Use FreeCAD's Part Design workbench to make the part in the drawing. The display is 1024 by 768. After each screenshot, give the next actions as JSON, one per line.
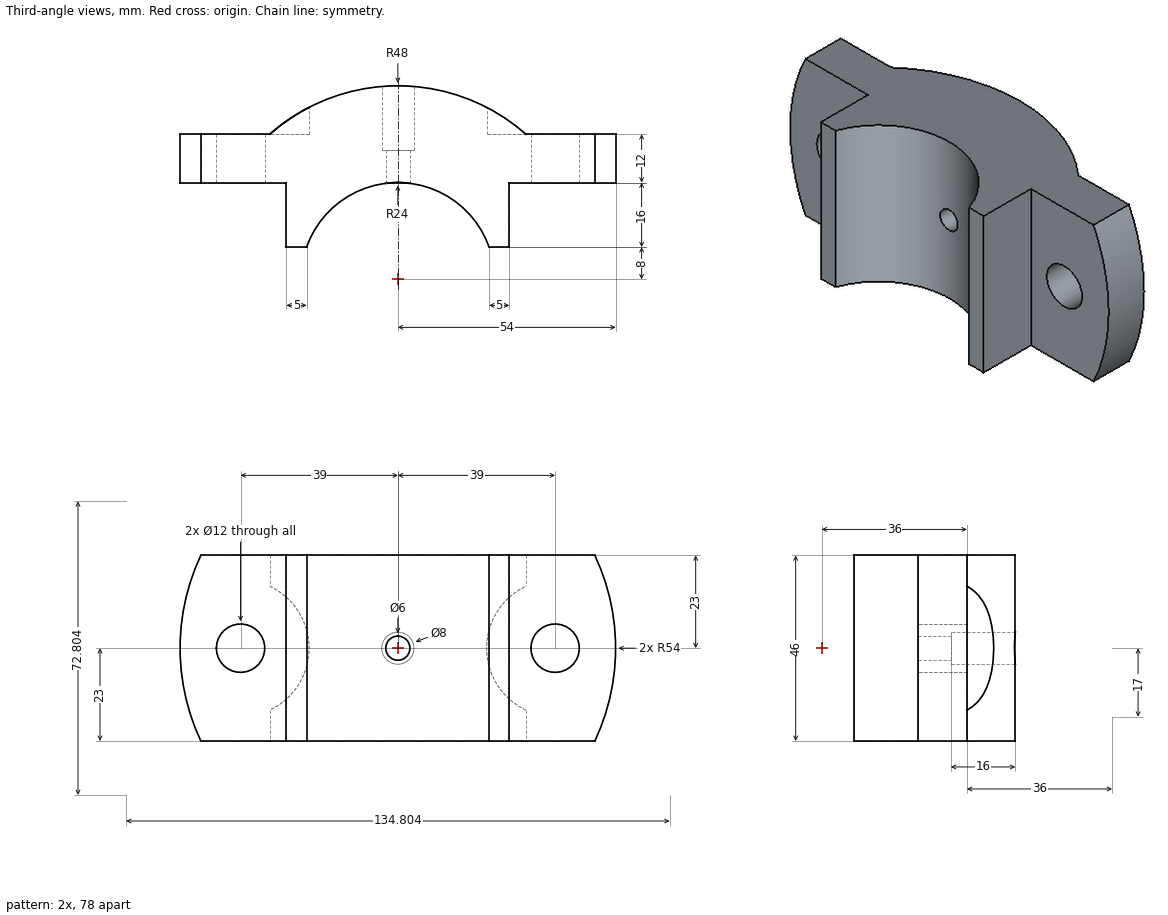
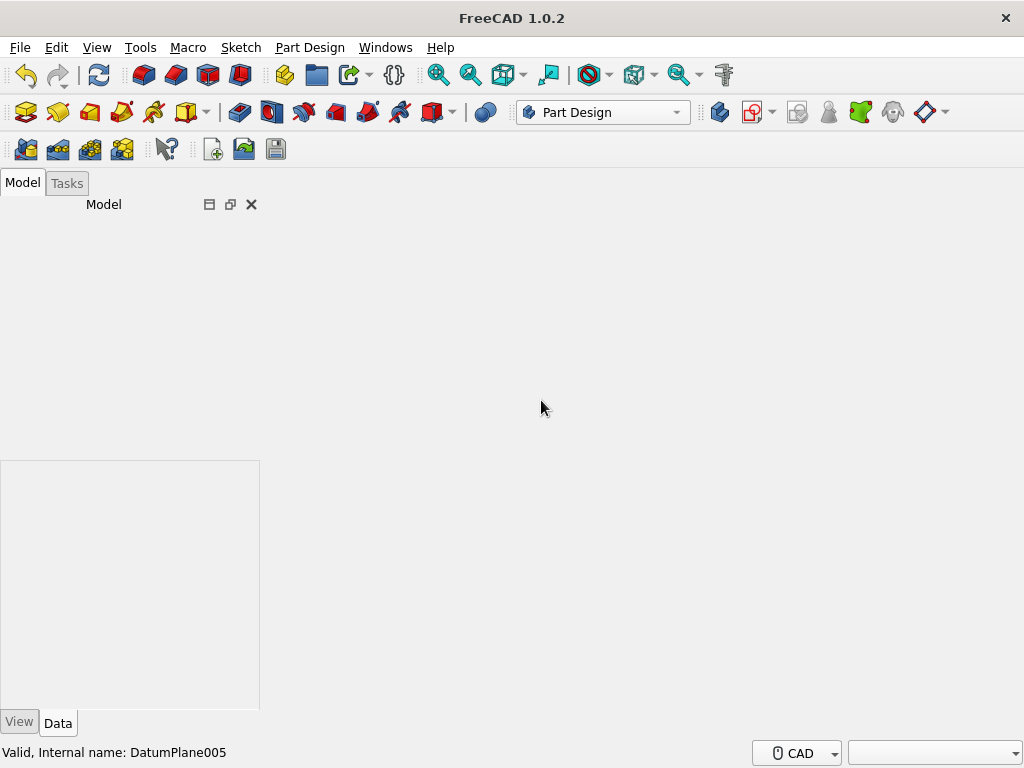
{"action": "left_click", "coordinate": [212, 150]}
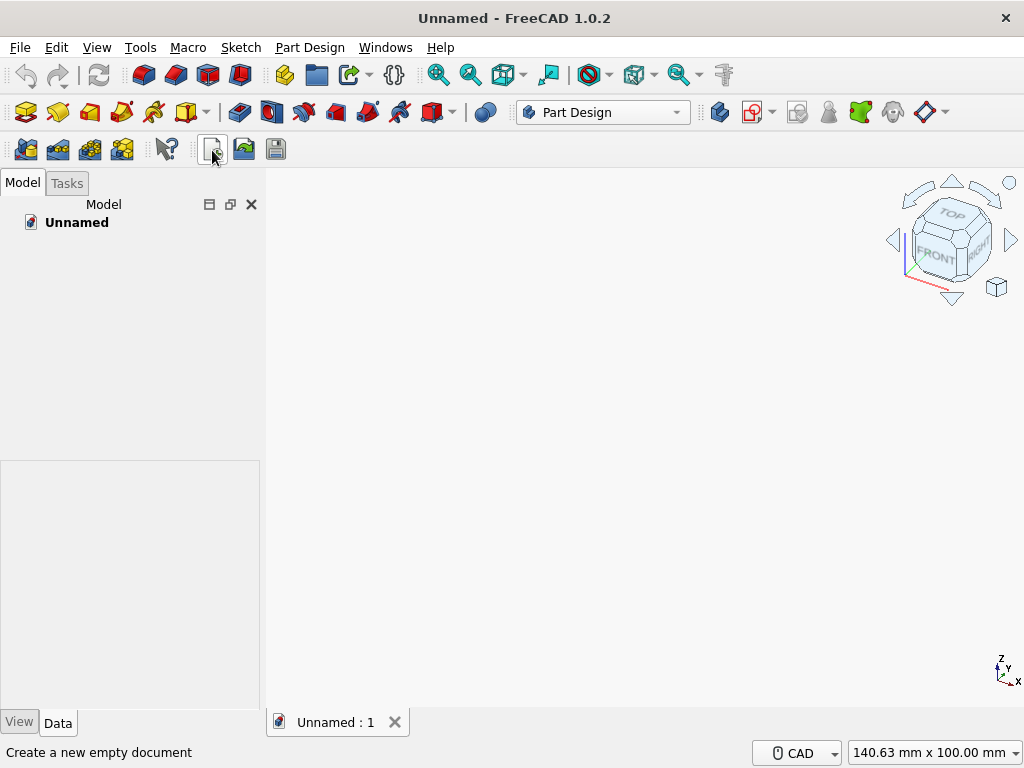
{"action": "left_click", "coordinate": [752, 112]}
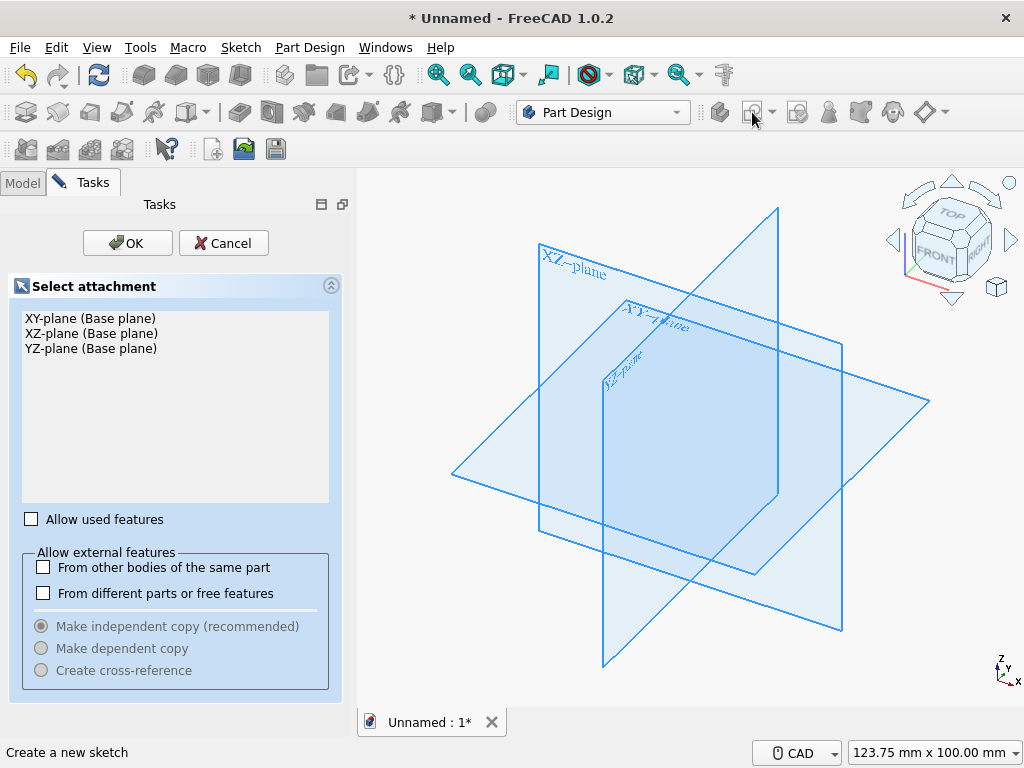
{"action": "left_click", "coordinate": [82, 318]}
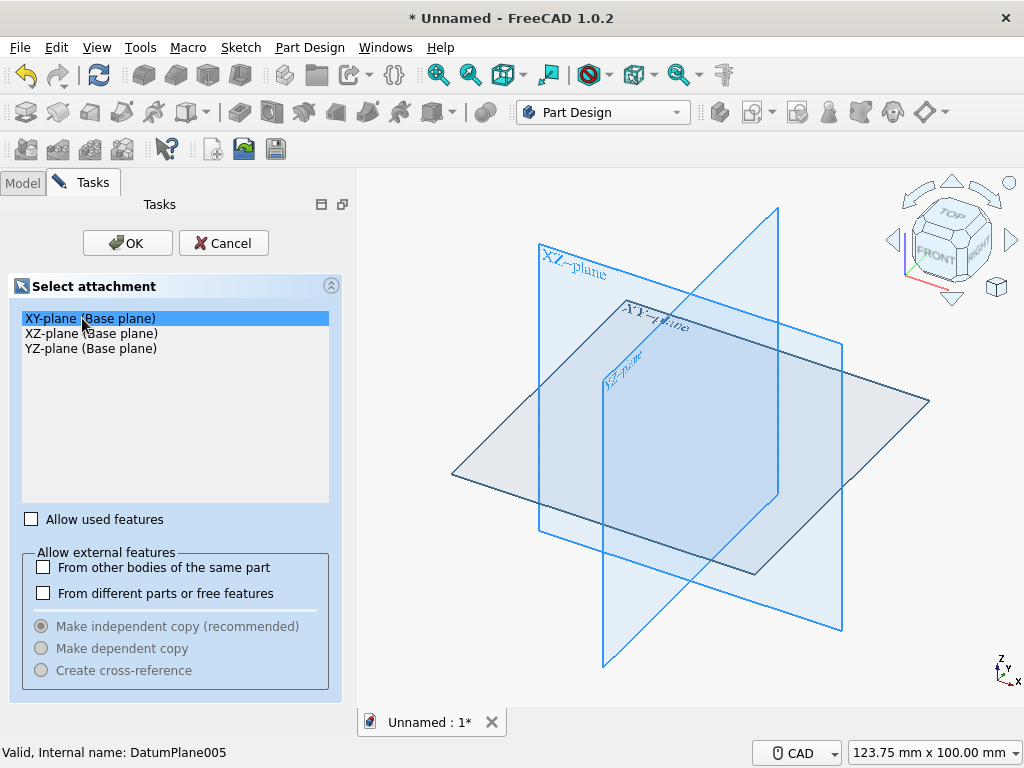
{"action": "left_click", "coordinate": [128, 243]}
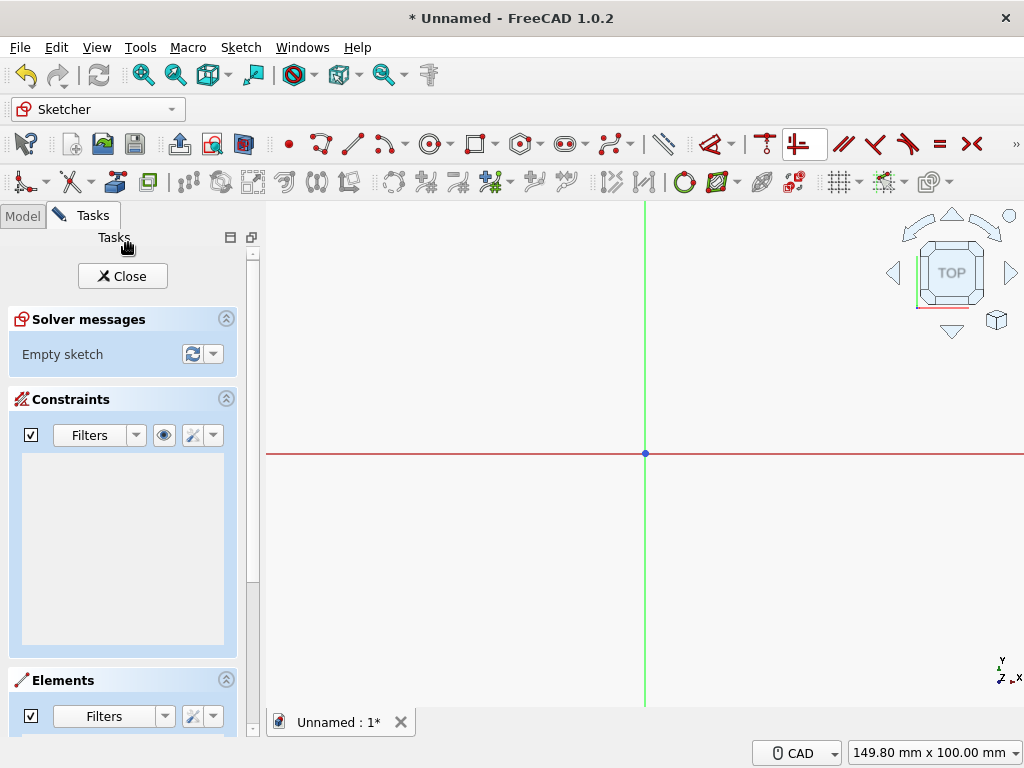
{"action": "scroll", "coordinate": [437, 679], "scroll_direction": "down", "scroll_amount": 2}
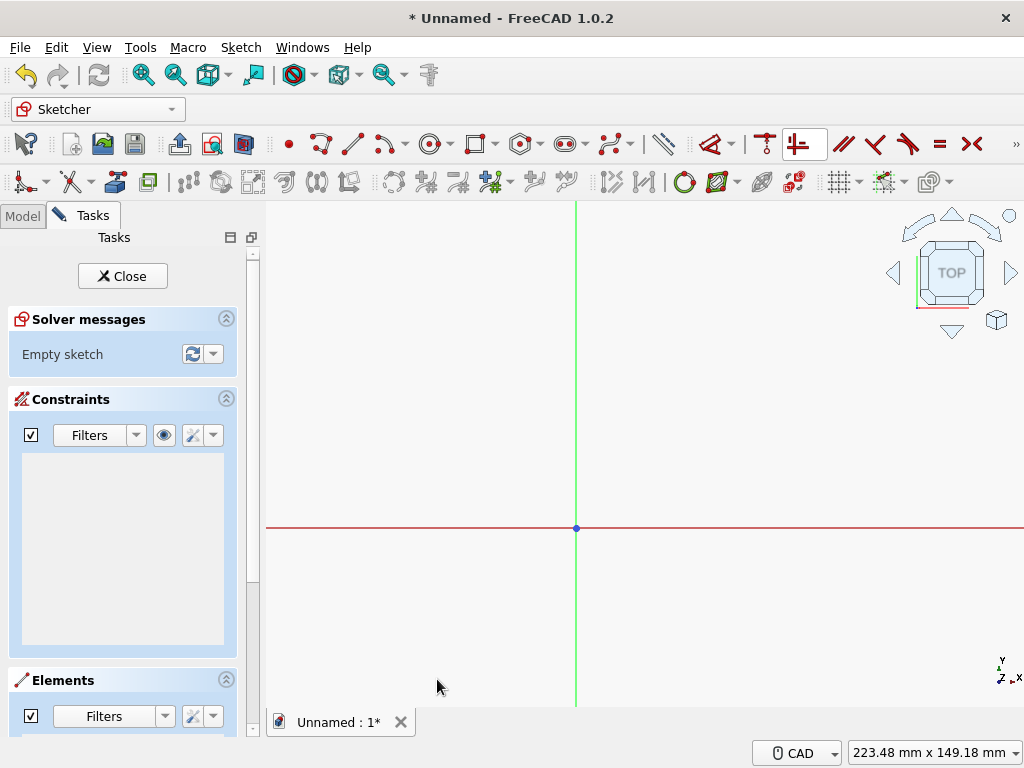
{"action": "left_click", "coordinate": [322, 144]}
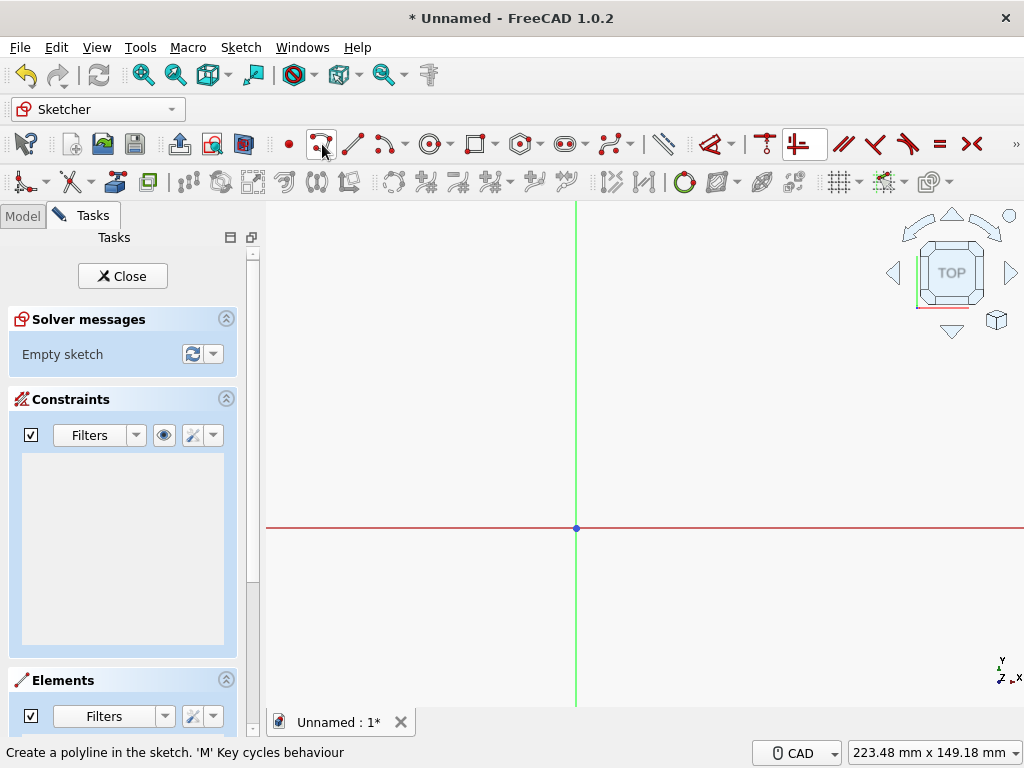
{"action": "left_click", "coordinate": [653, 501]}
{"action": "left_click", "coordinate": [670, 501]}
{"action": "left_click", "coordinate": [670, 447]}
{"action": "left_click", "coordinate": [760, 447]}
{"action": "left_click", "coordinate": [760, 406]}
{"action": "left_click", "coordinate": [684, 406]}
{"action": "right_click", "coordinate": [684, 406]}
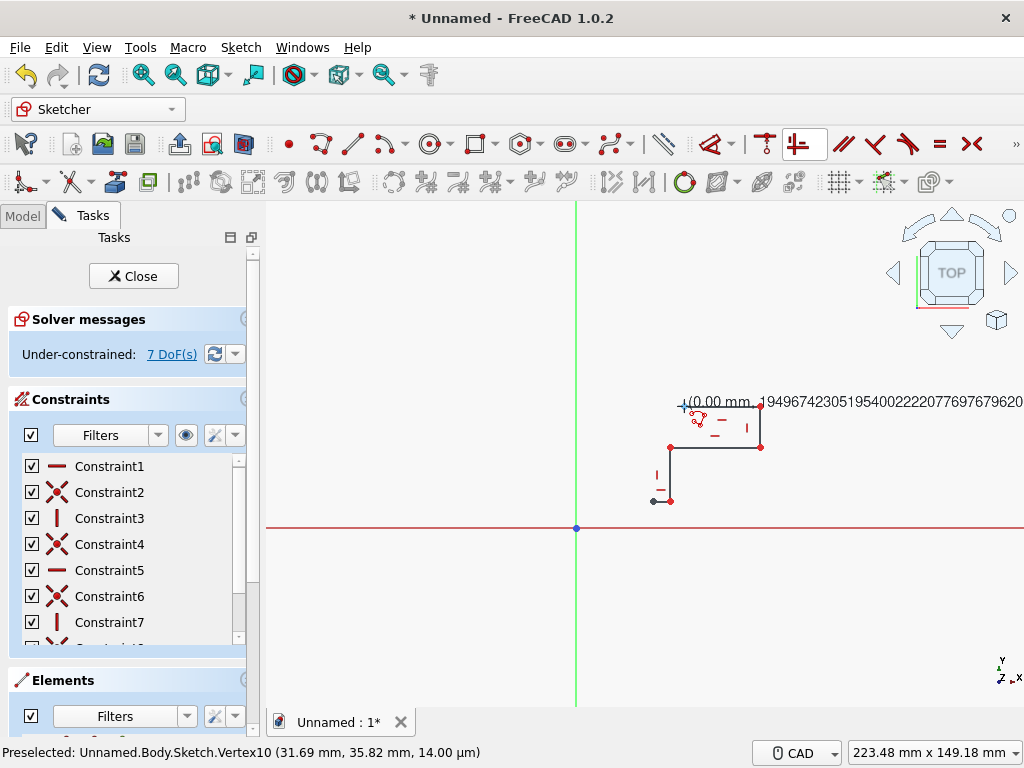
{"action": "left_click", "coordinate": [469, 406]}
{"action": "left_click", "coordinate": [393, 406]}
{"action": "left_click", "coordinate": [393, 447]}
{"action": "left_click", "coordinate": [483, 447]}
{"action": "left_click", "coordinate": [483, 501]}
{"action": "left_click", "coordinate": [500, 501]}
{"action": "right_click", "coordinate": [500, 501]}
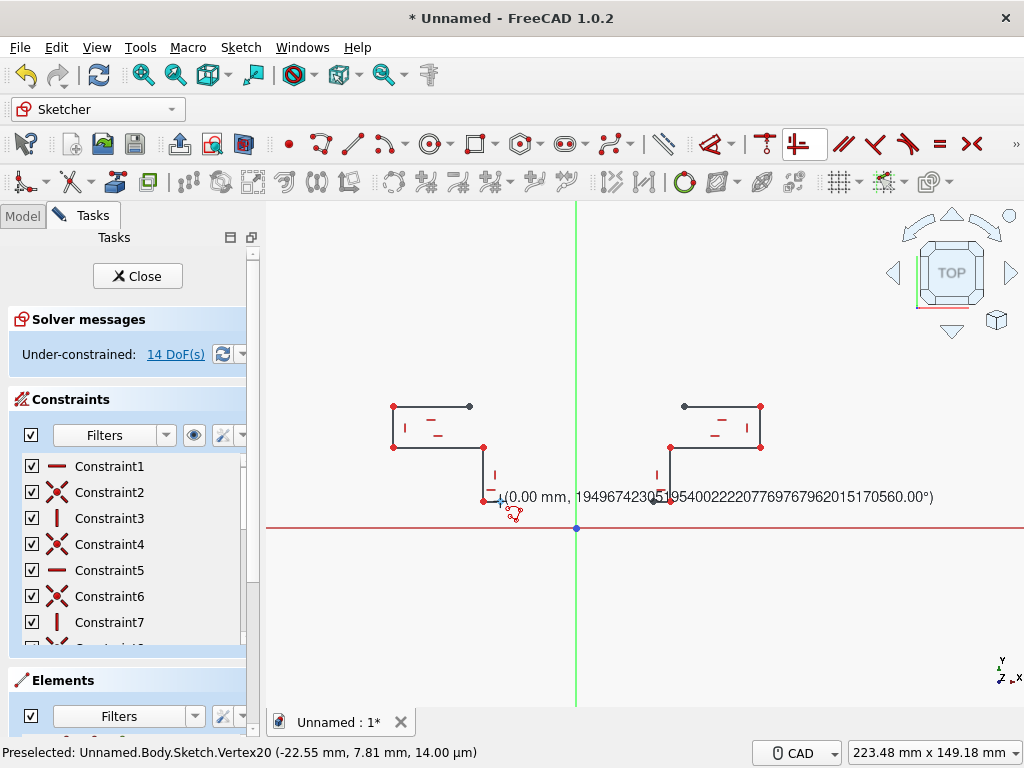
{"action": "key", "text": "g 3 a"}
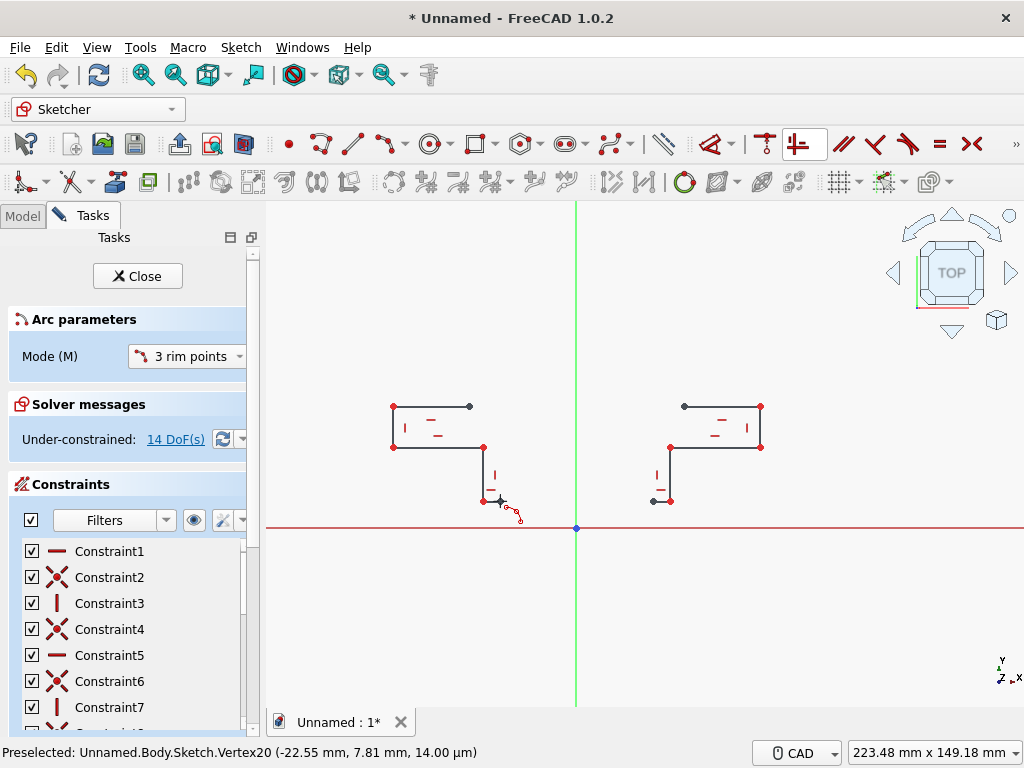
{"action": "left_click", "coordinate": [684, 407]}
{"action": "left_click", "coordinate": [469, 407]}
{"action": "left_click", "coordinate": [600, 367]}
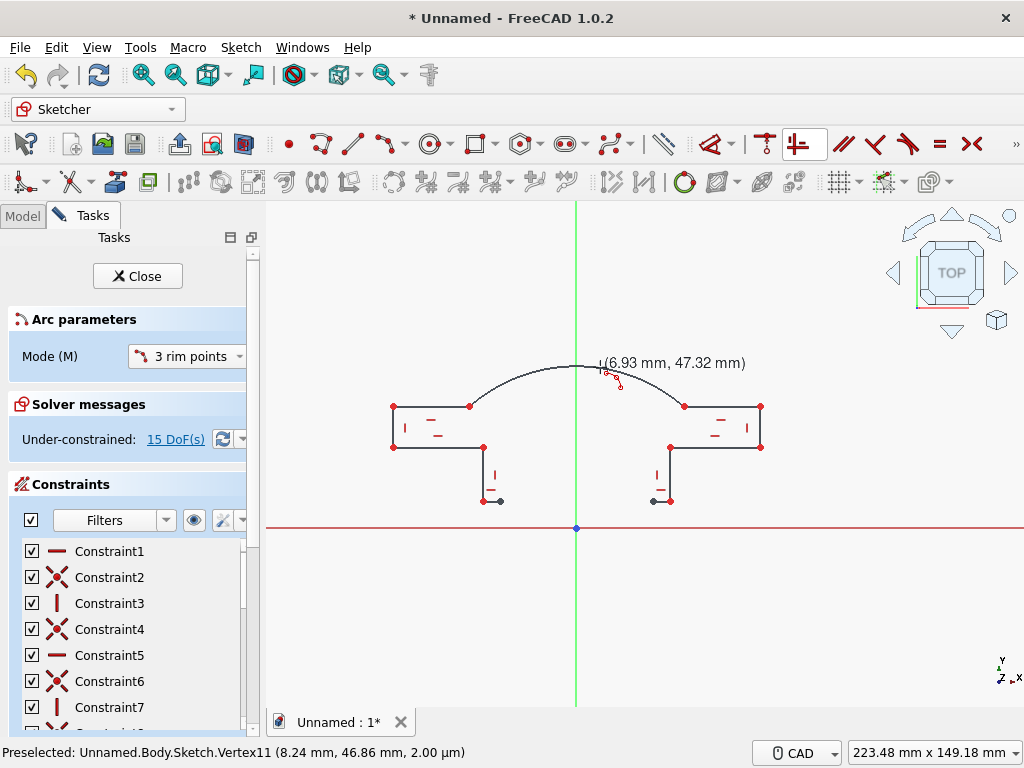
{"action": "scroll", "coordinate": [500, 501], "scroll_direction": "up", "scroll_amount": 4}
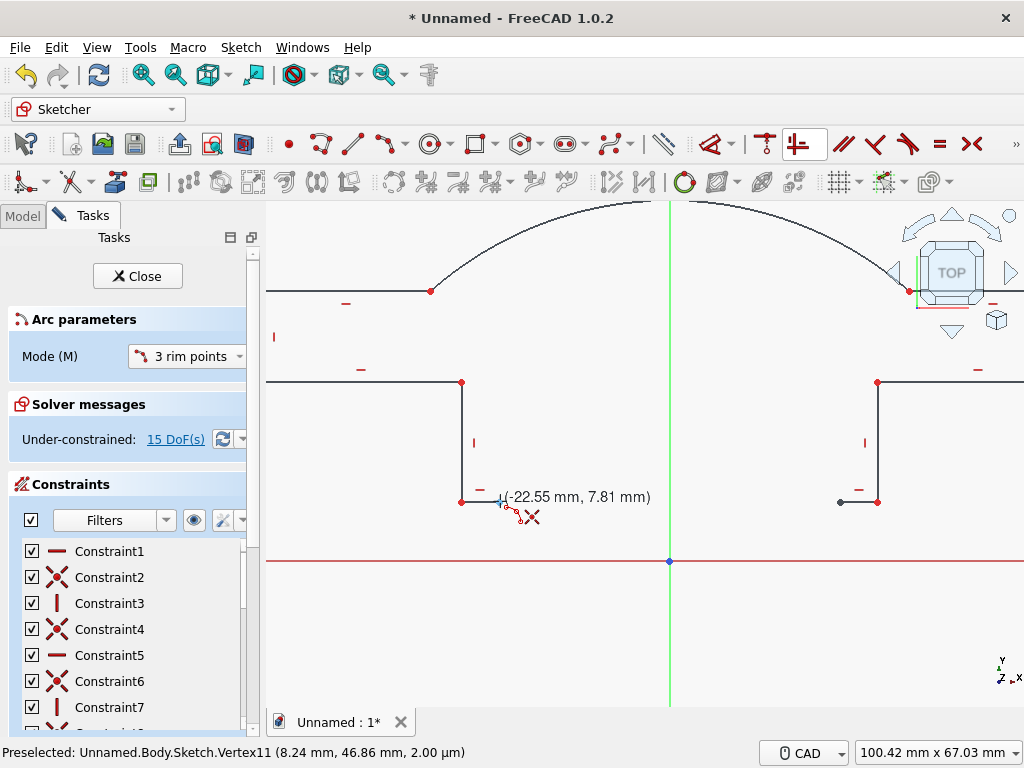
{"action": "left_click", "coordinate": [500, 502]}
{"action": "left_click", "coordinate": [840, 502]}
{"action": "left_click", "coordinate": [714, 386]}
{"action": "key", "text": "Escape"}